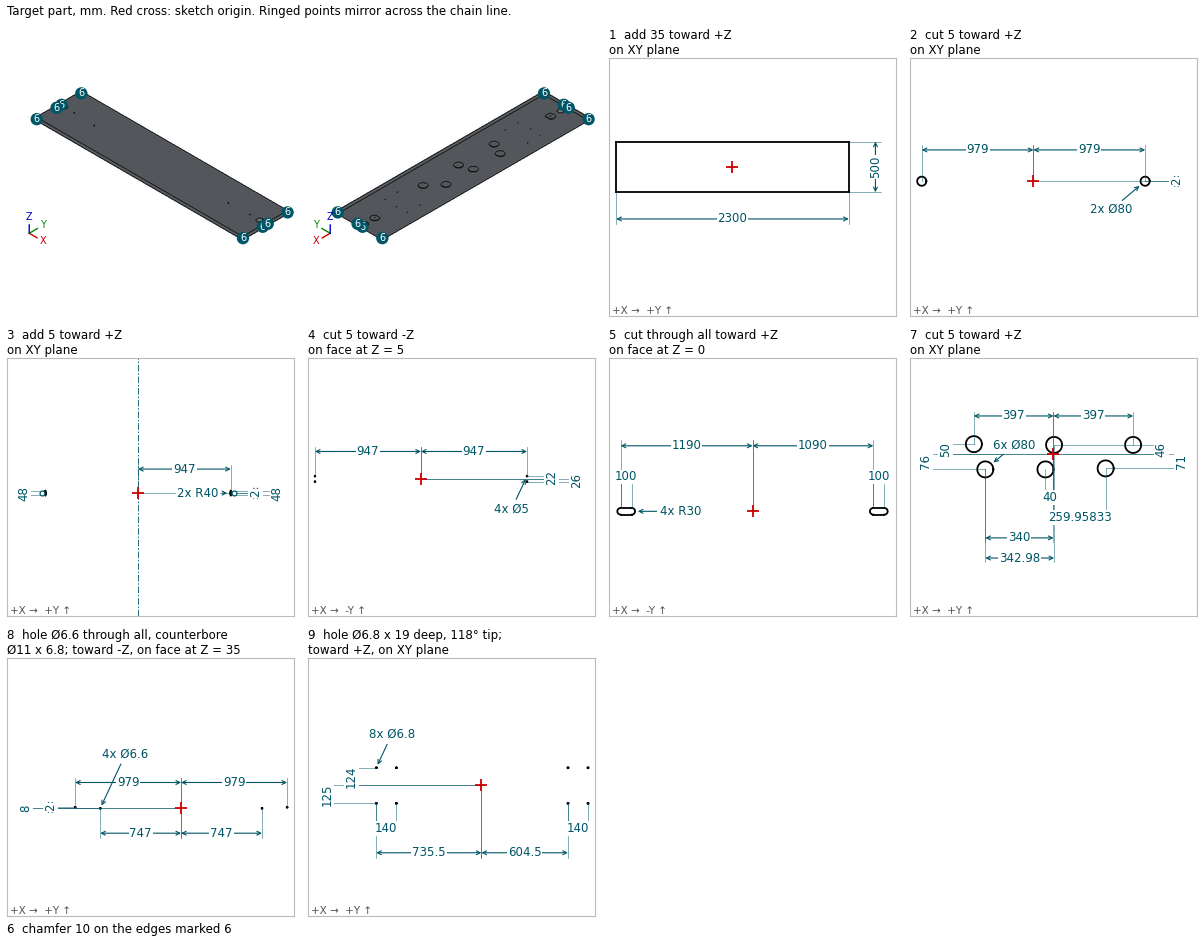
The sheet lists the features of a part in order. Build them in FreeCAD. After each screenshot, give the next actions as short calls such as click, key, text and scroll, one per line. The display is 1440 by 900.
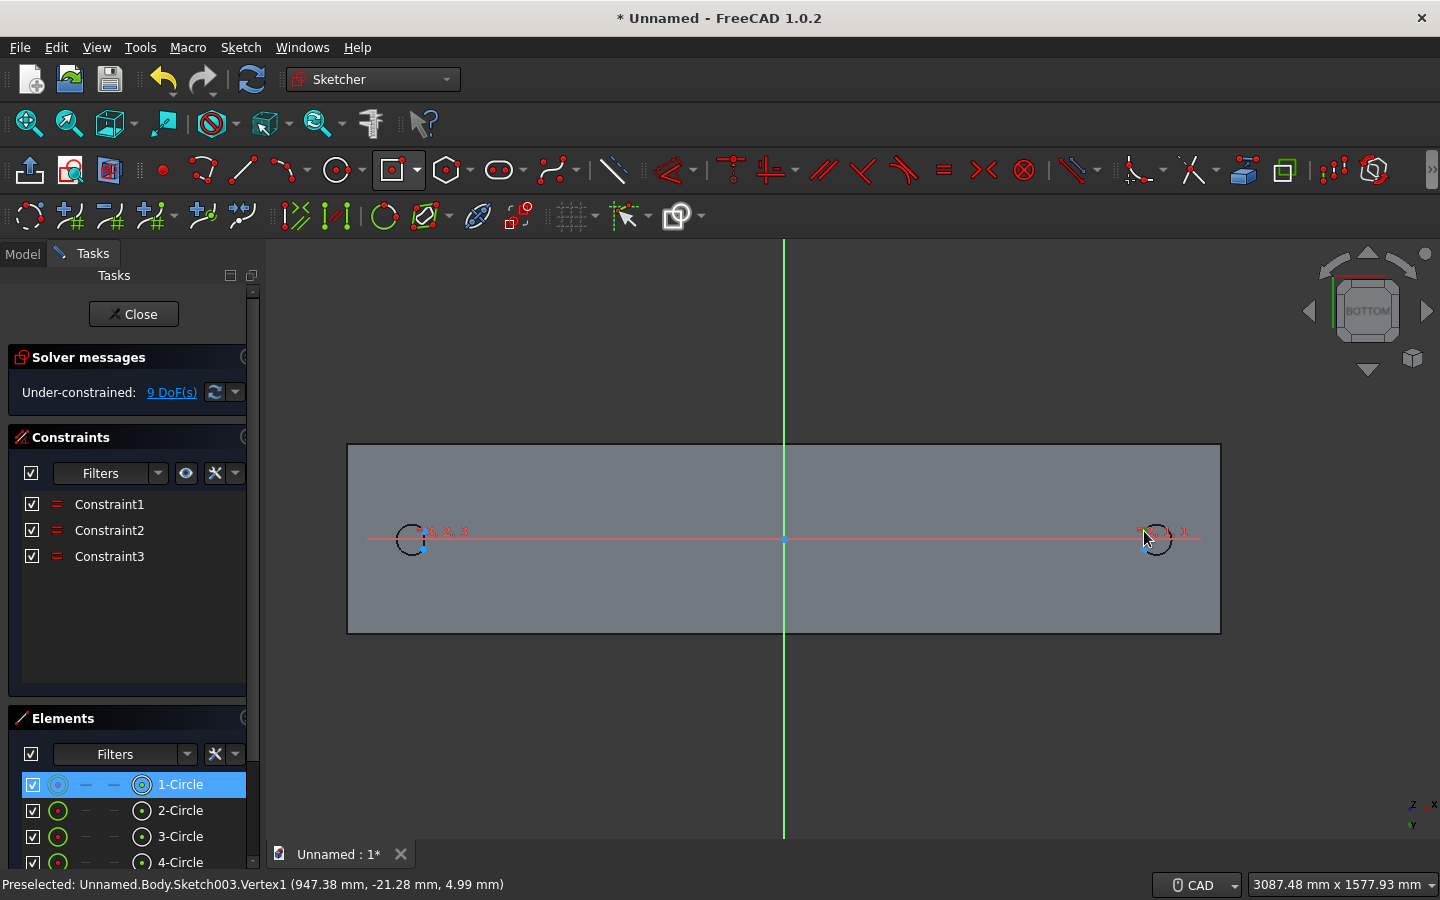
click(1144, 549)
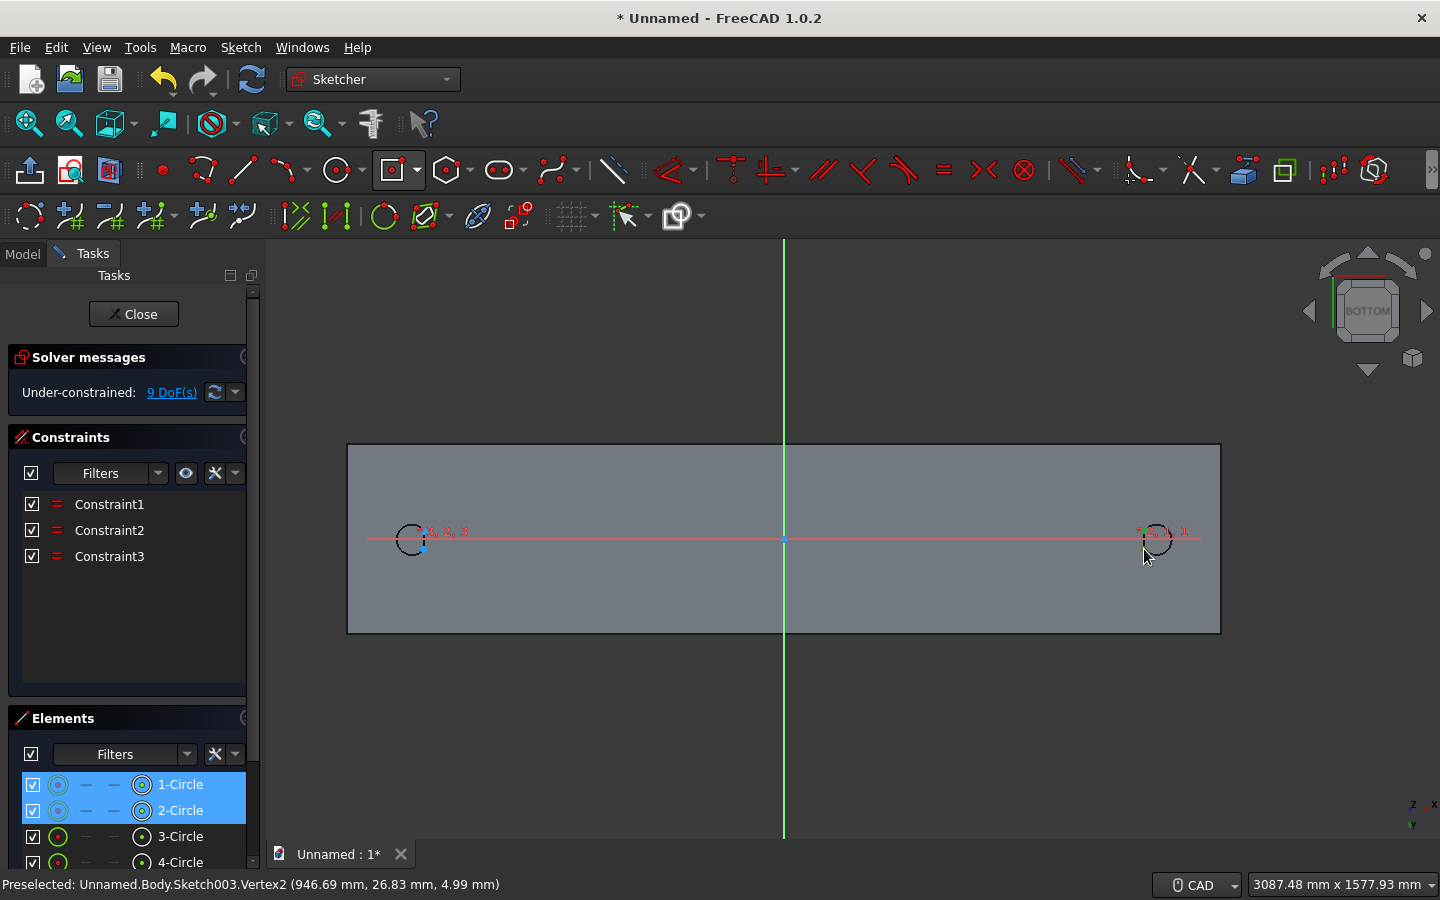
key(v)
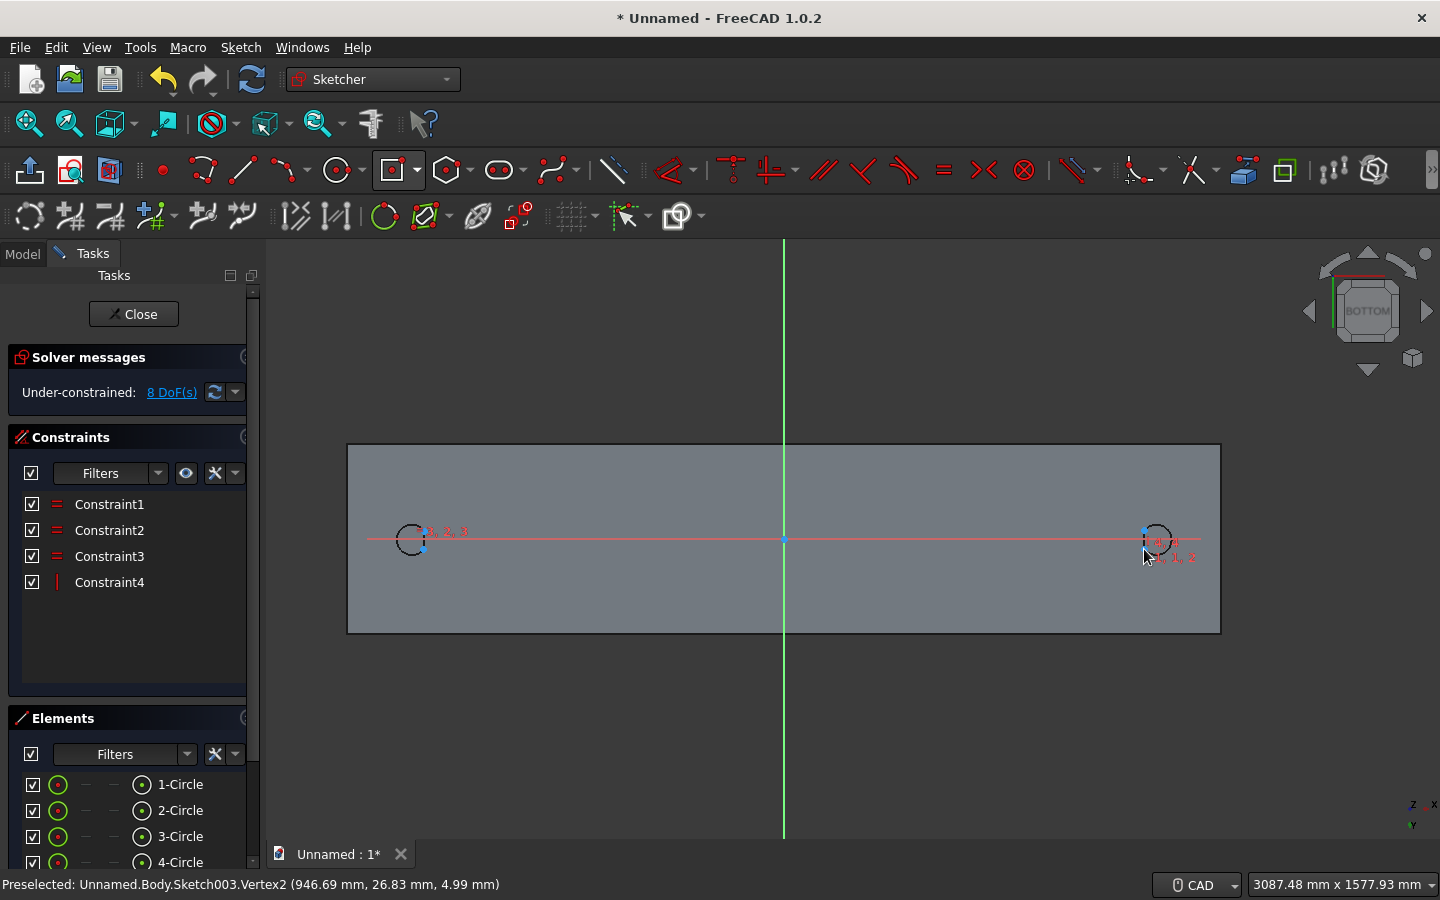
click(1144, 531)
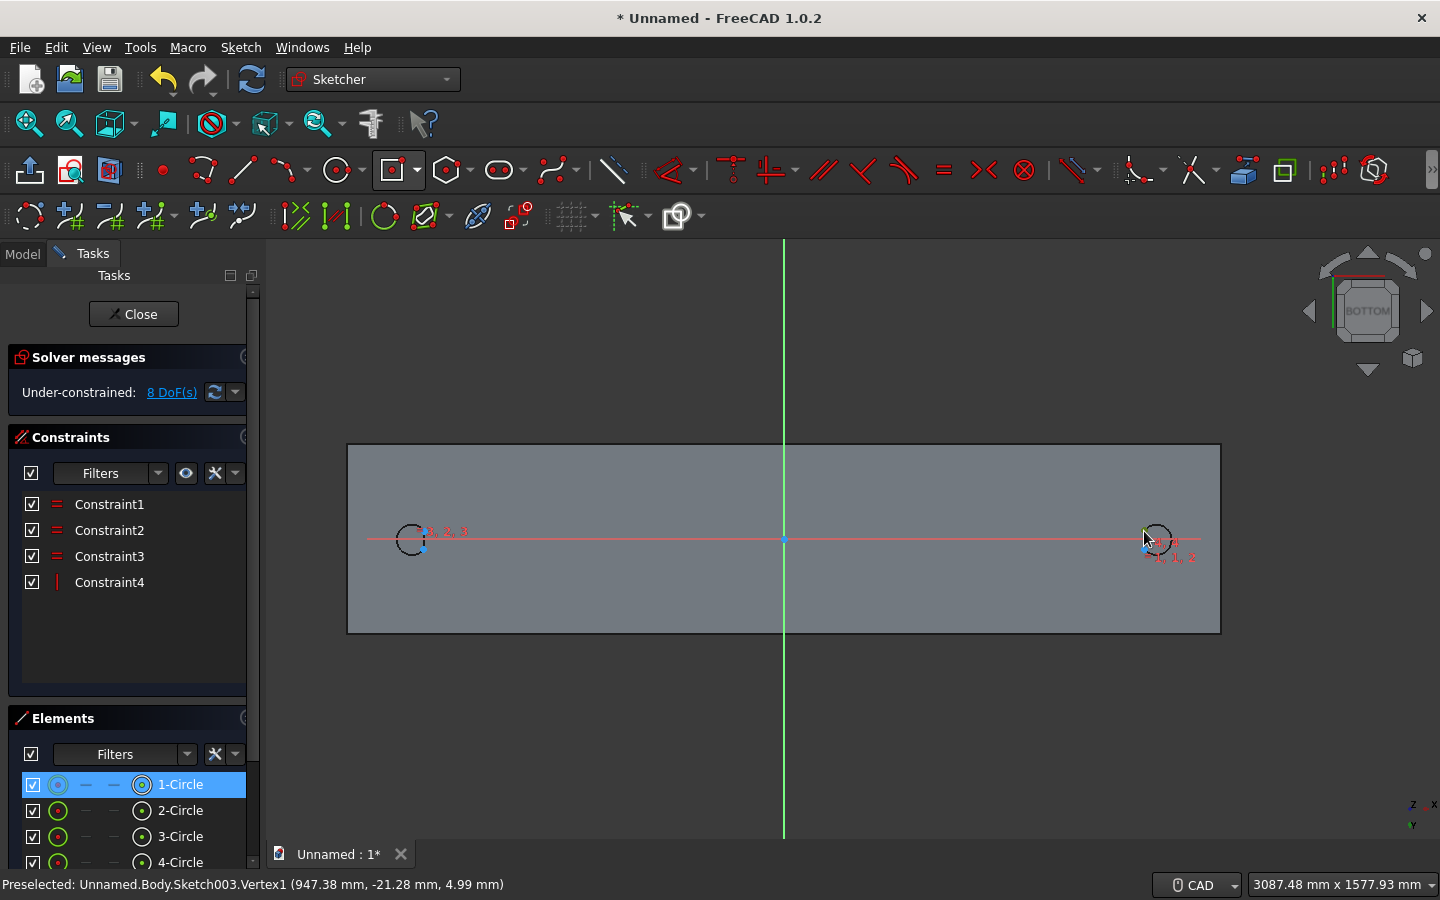
scroll(424, 531, up, 4)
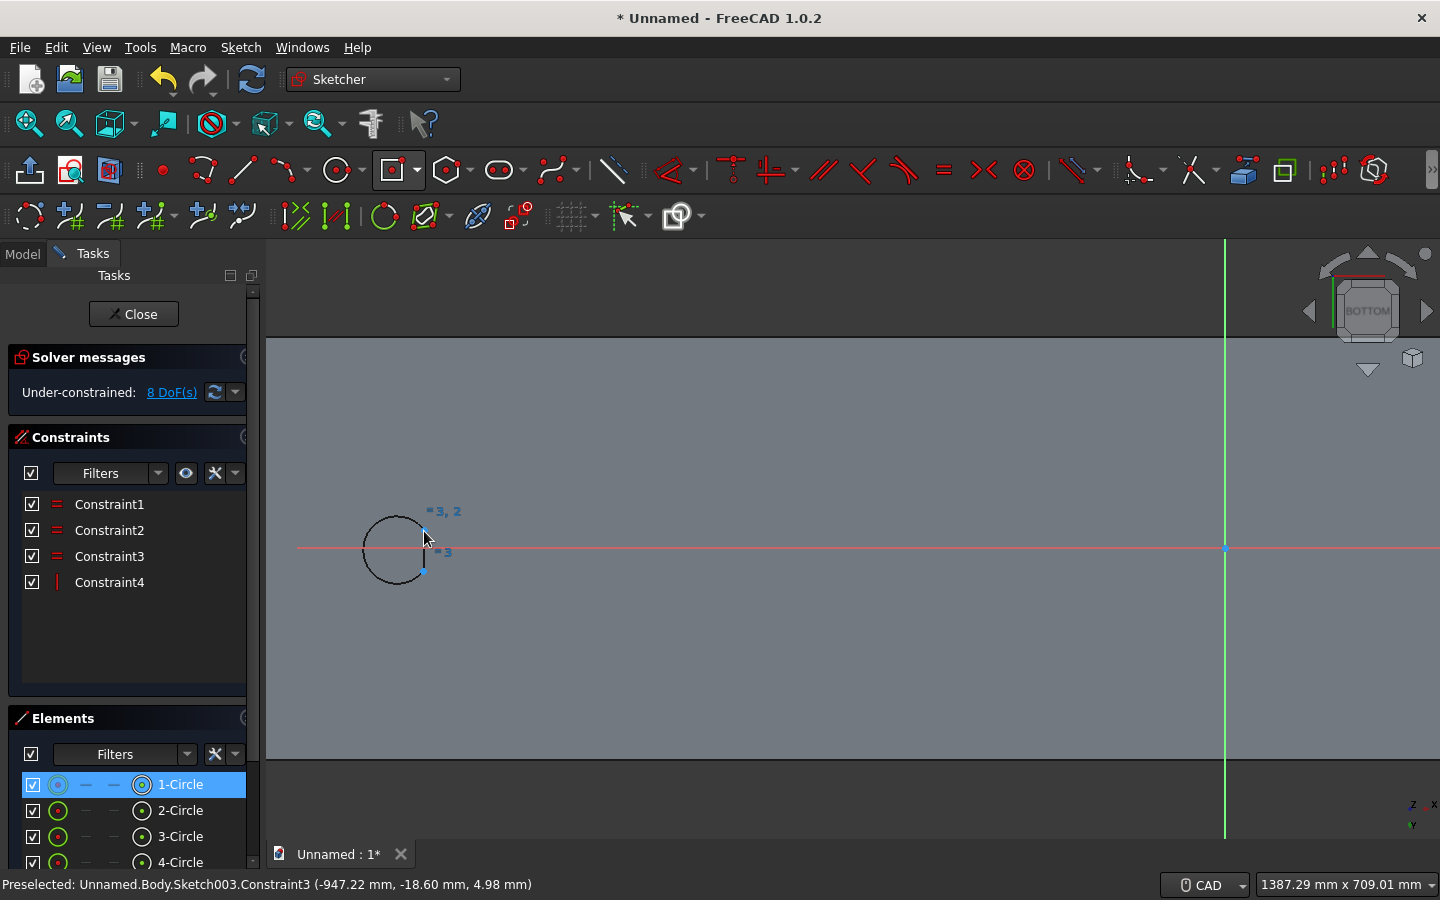
click(424, 531)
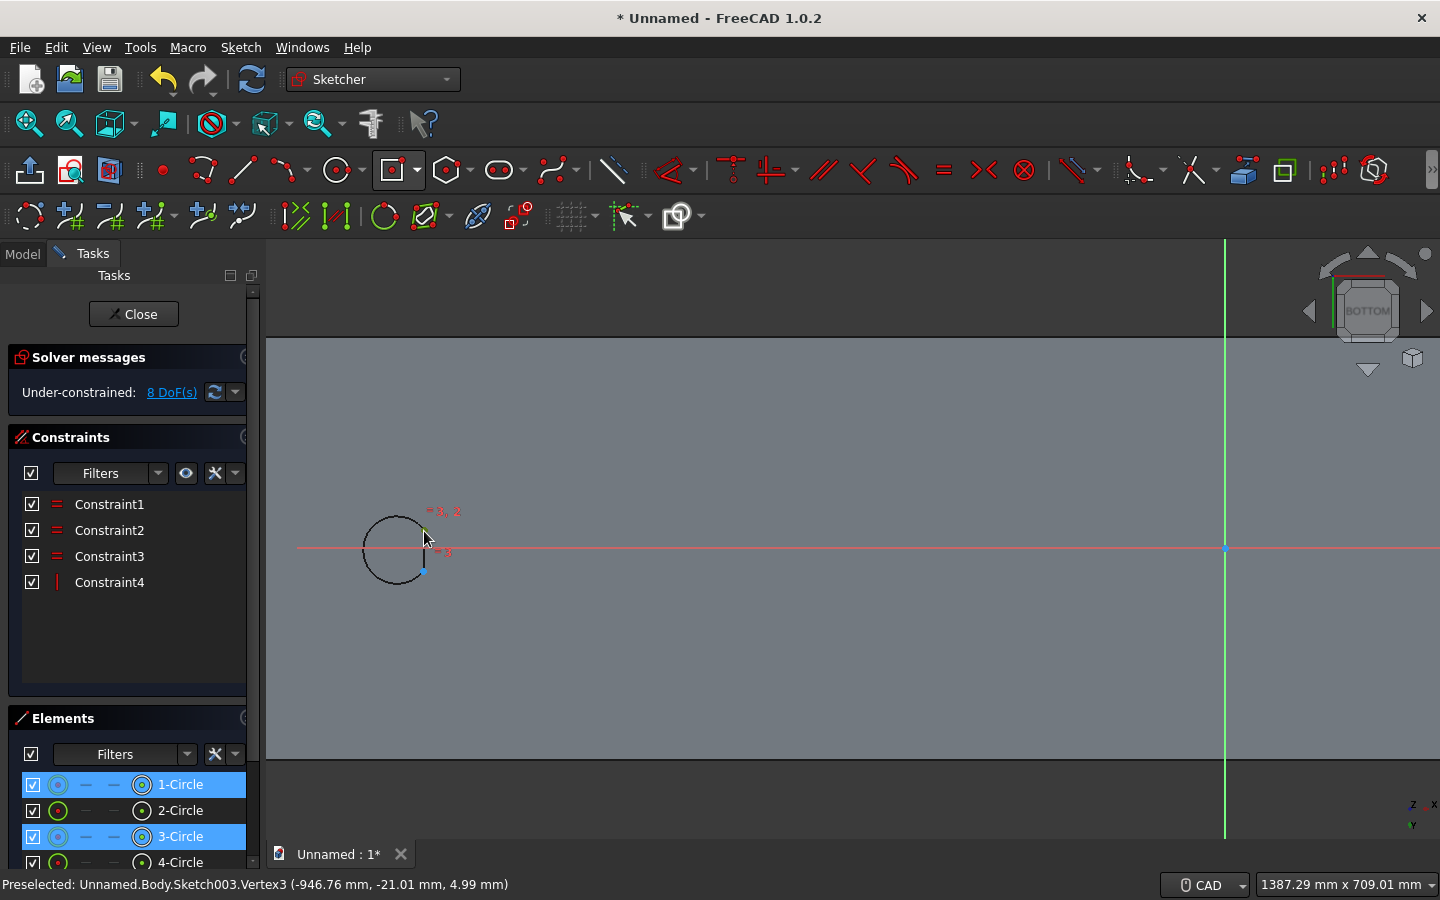
key(h)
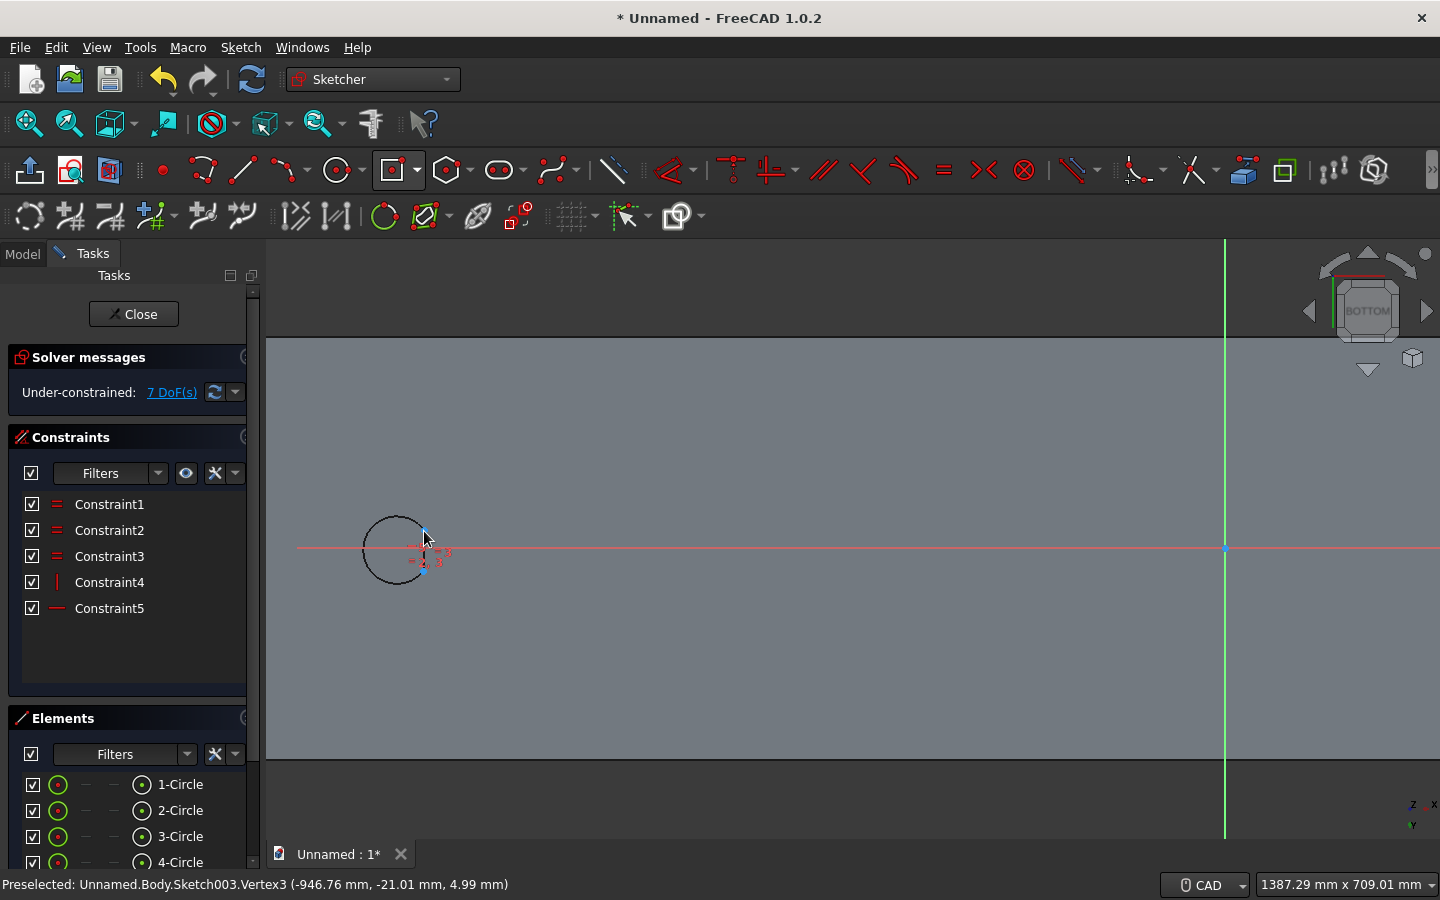
click(424, 530)